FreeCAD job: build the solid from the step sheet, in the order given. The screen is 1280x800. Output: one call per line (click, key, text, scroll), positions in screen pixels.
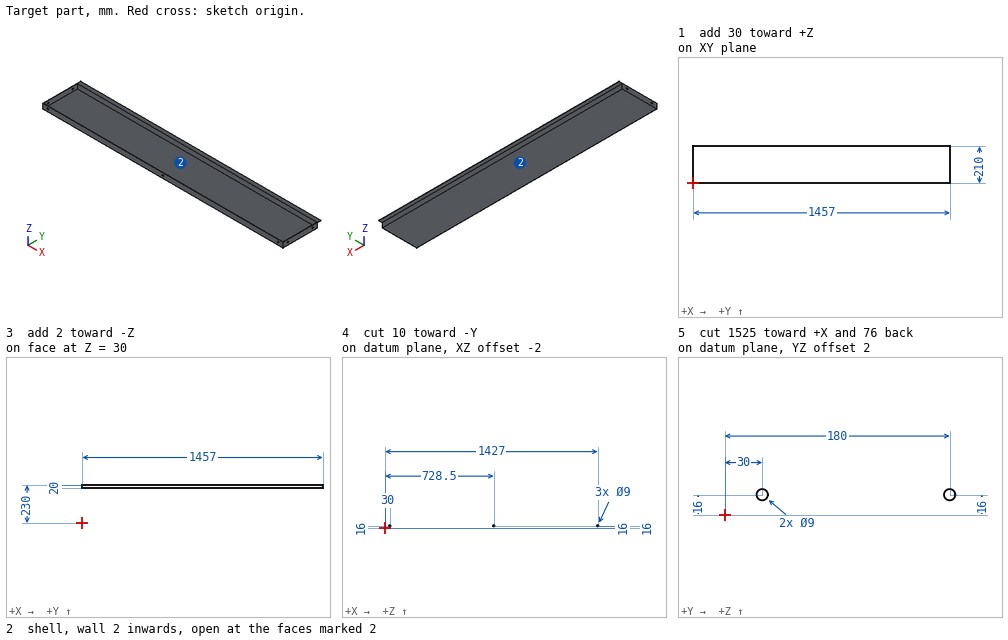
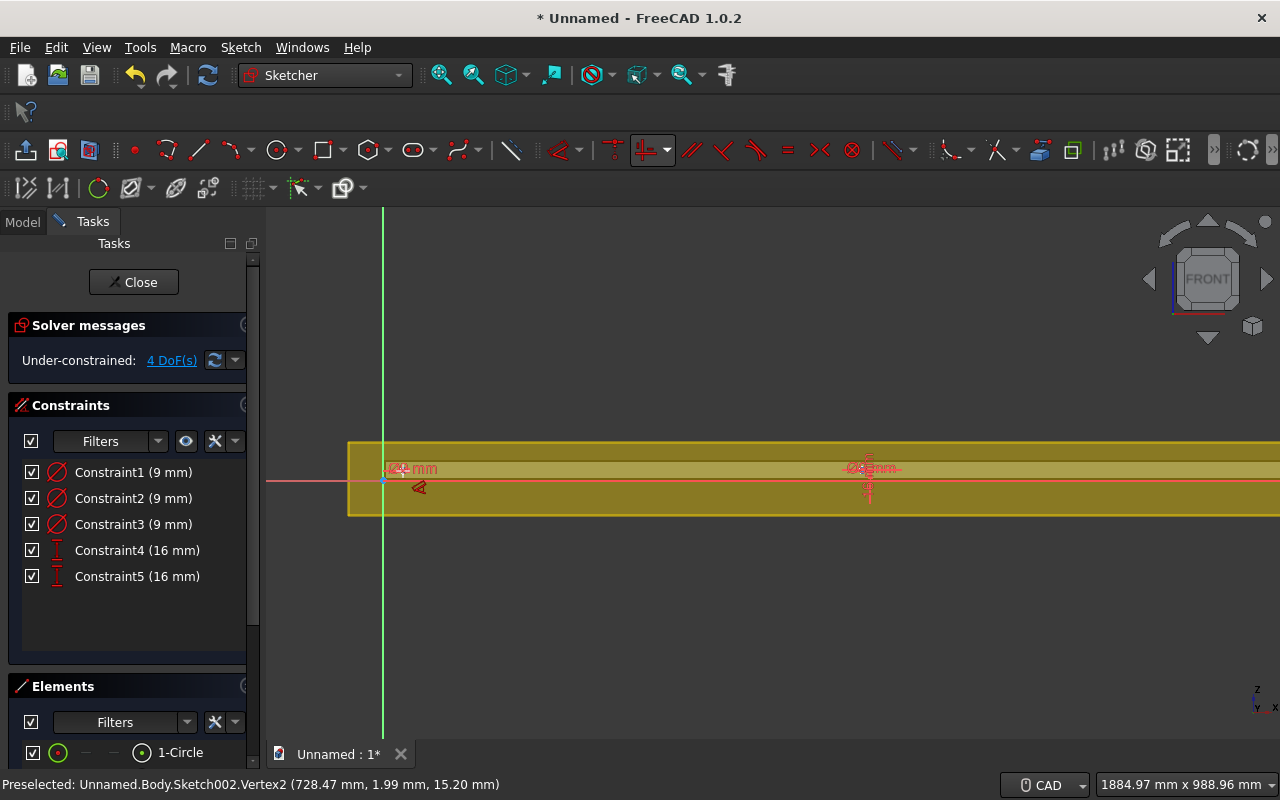
click(404, 470)
click(381, 526)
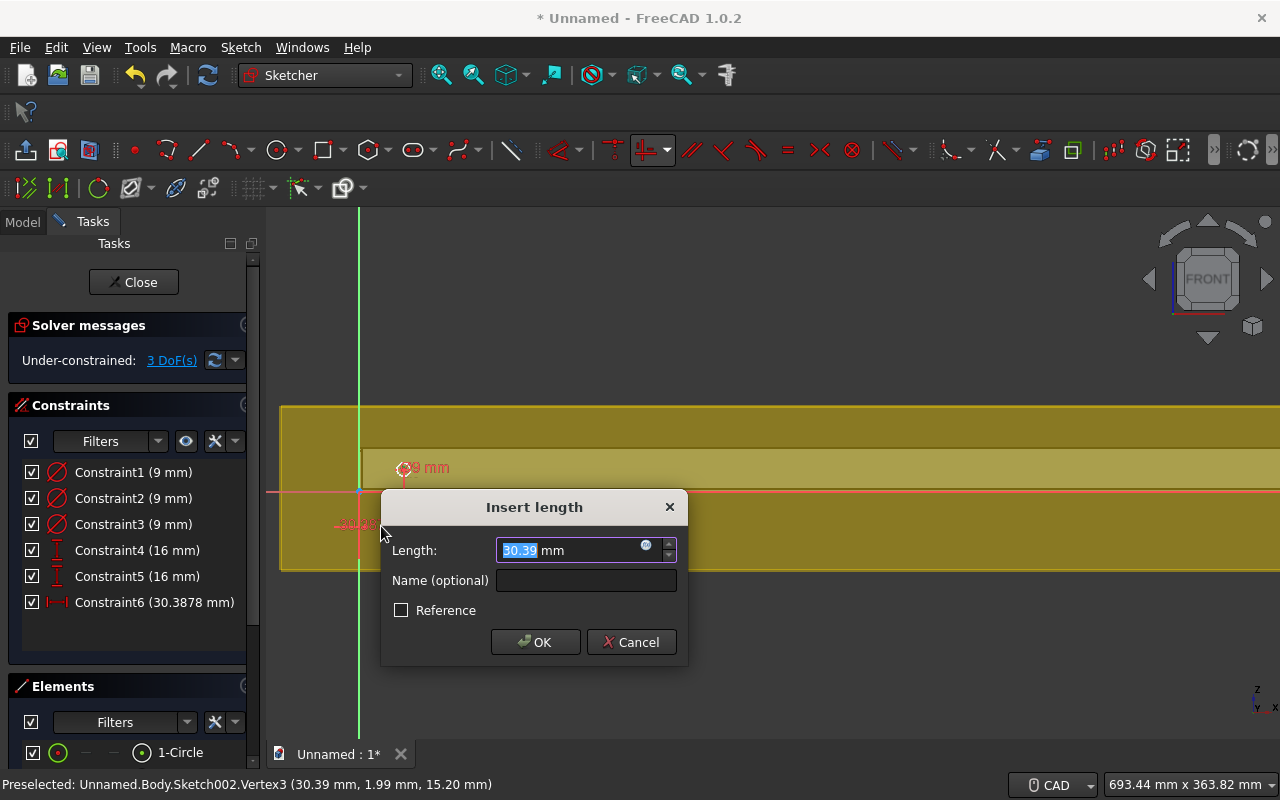
text(30)
key(Return)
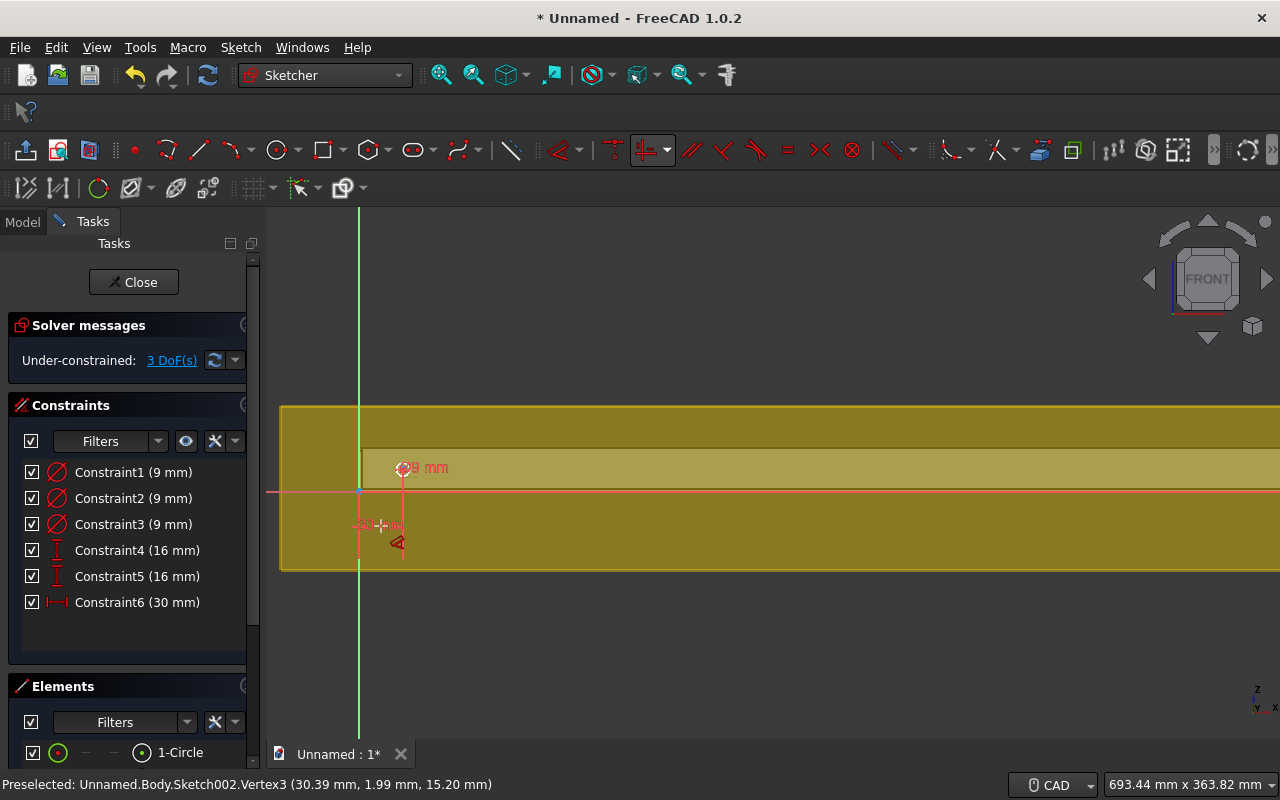
scroll(403, 470, up, 3)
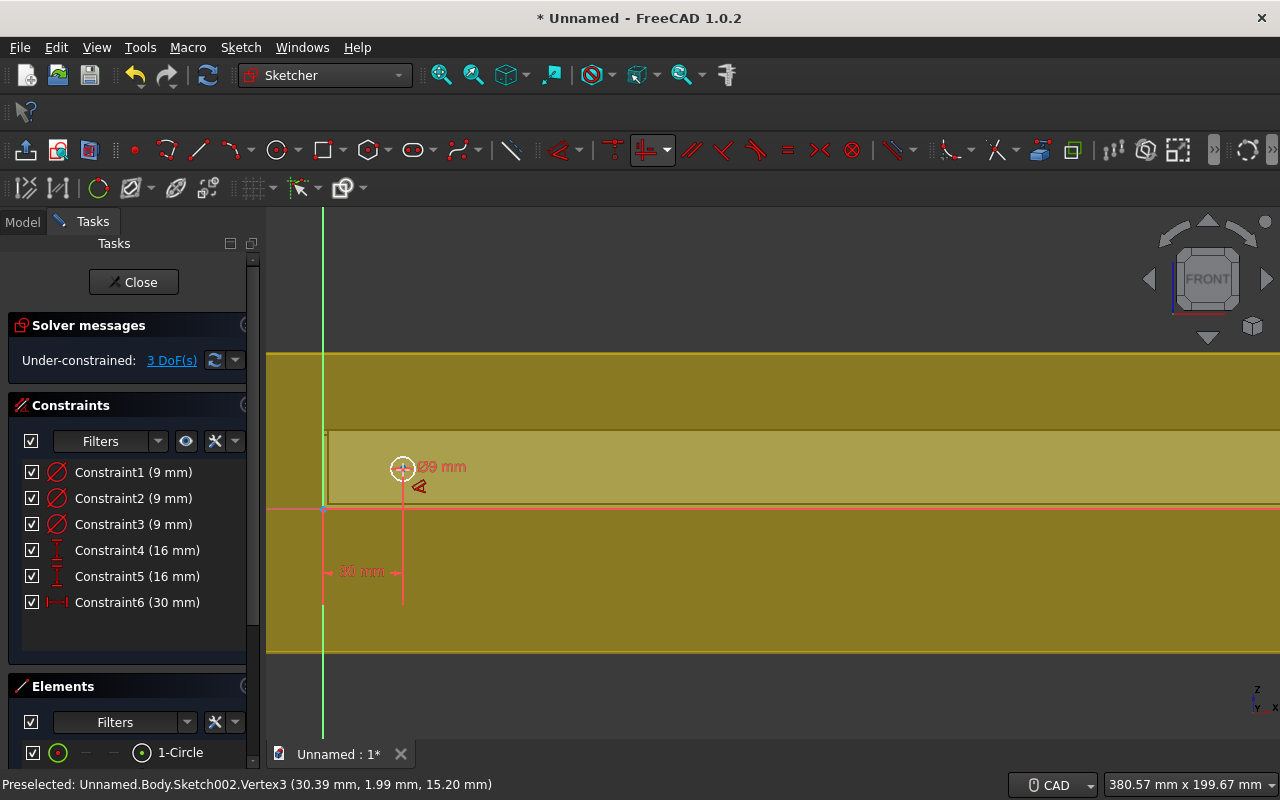
click(403, 469)
click(437, 489)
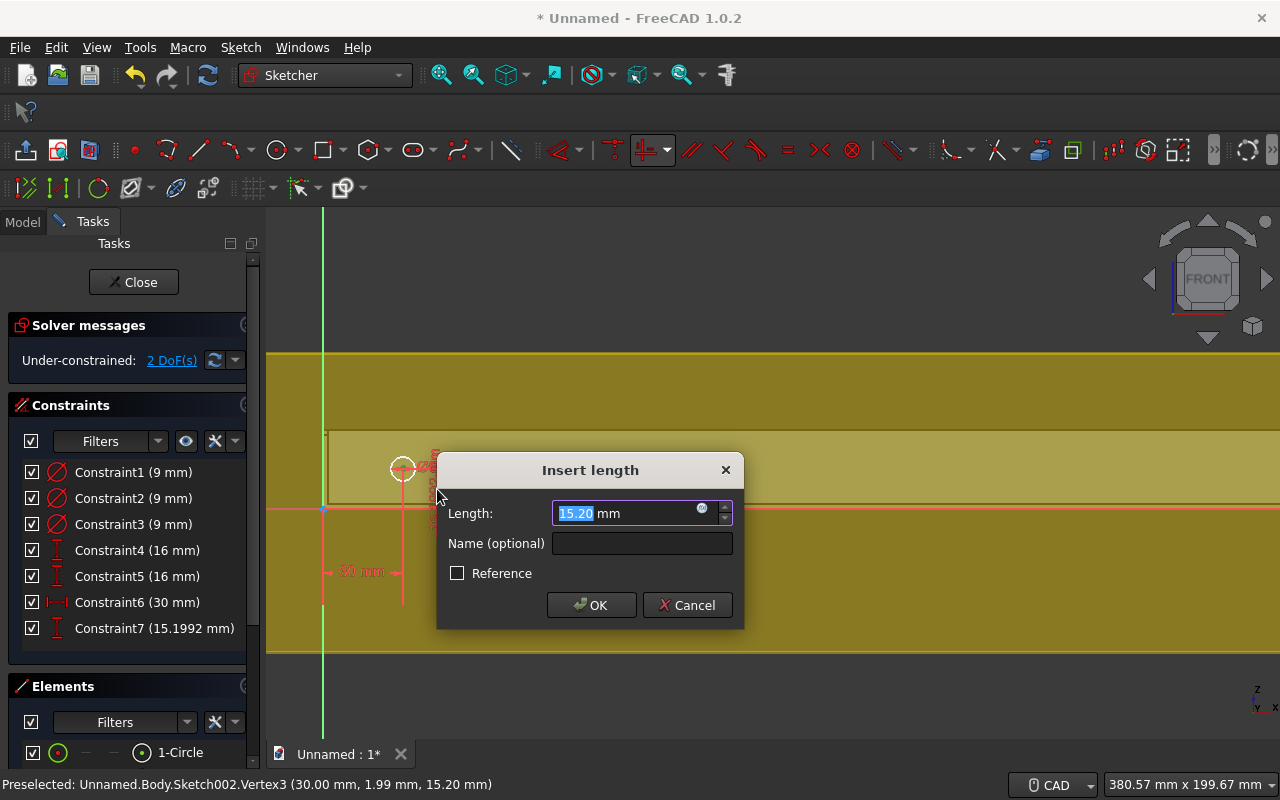
text(16)
key(Return)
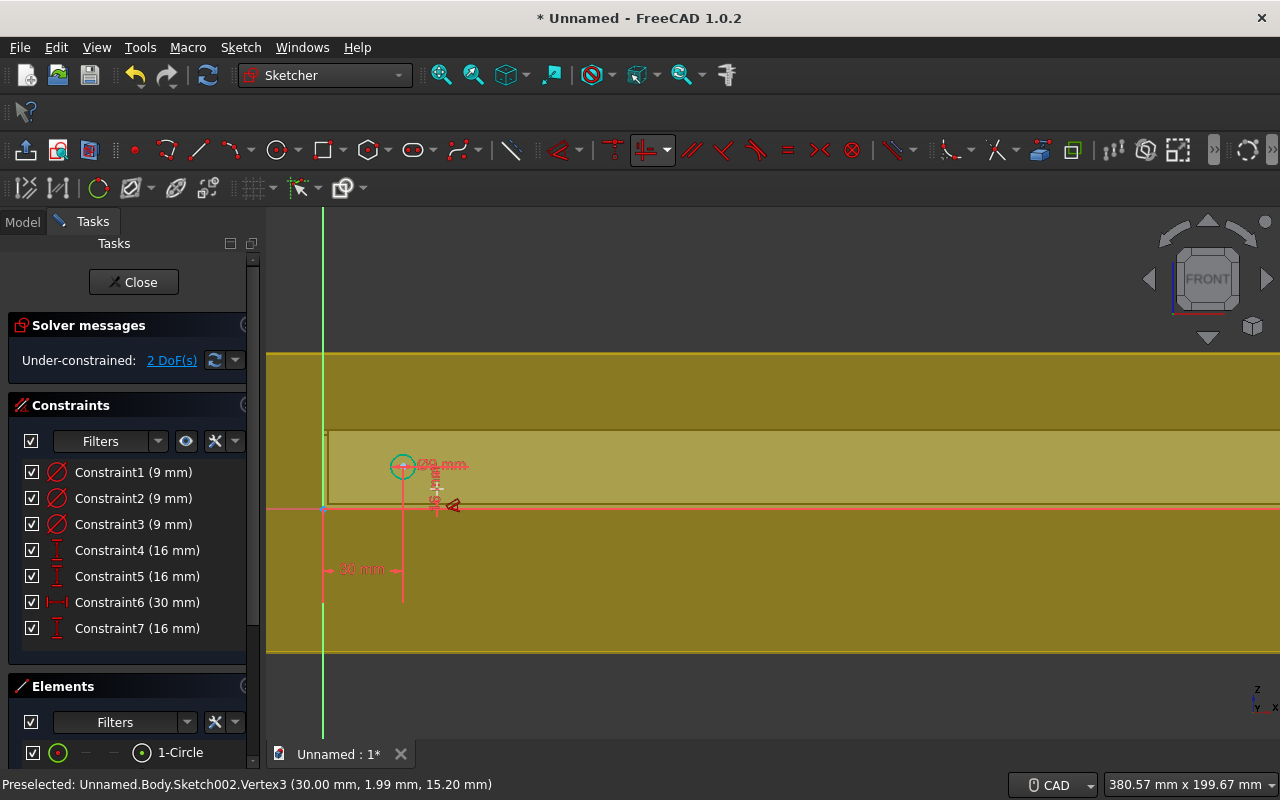
scroll(402, 471, down, 9)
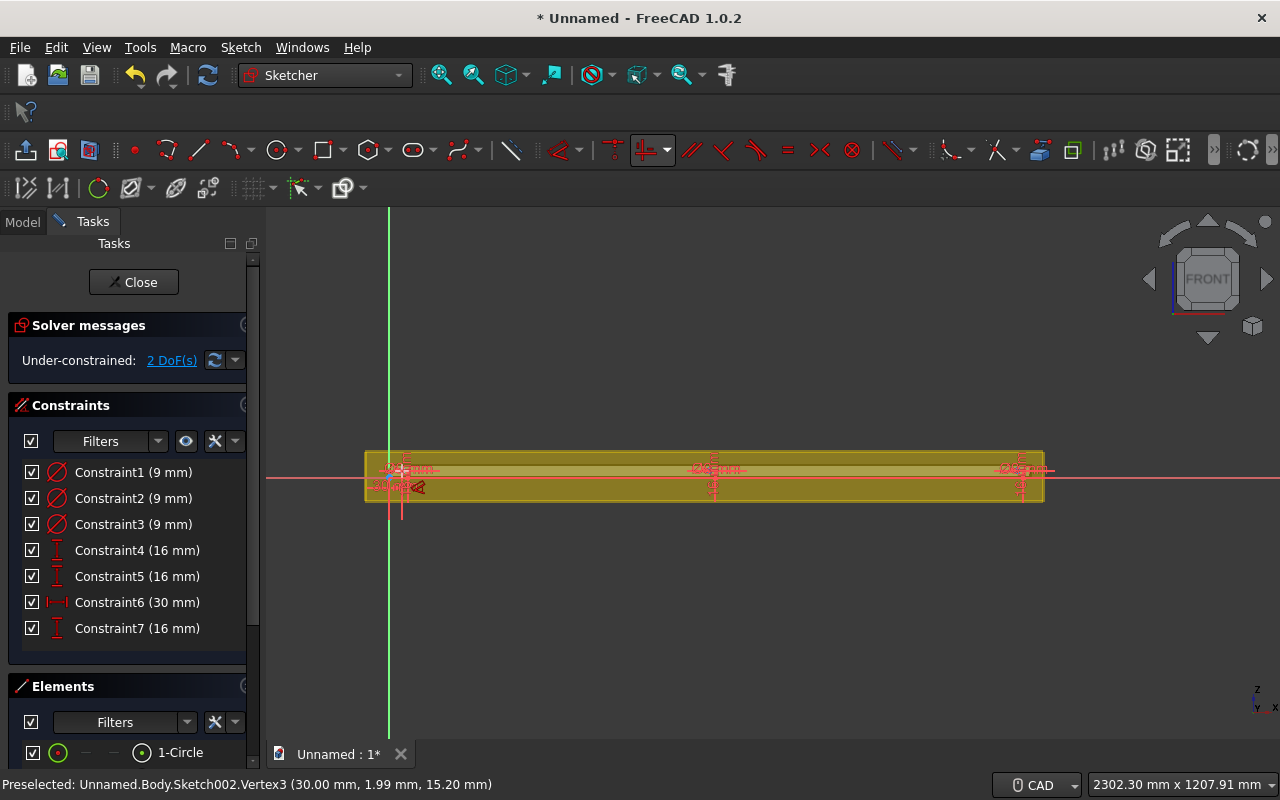
click(1017, 471)
click(703, 512)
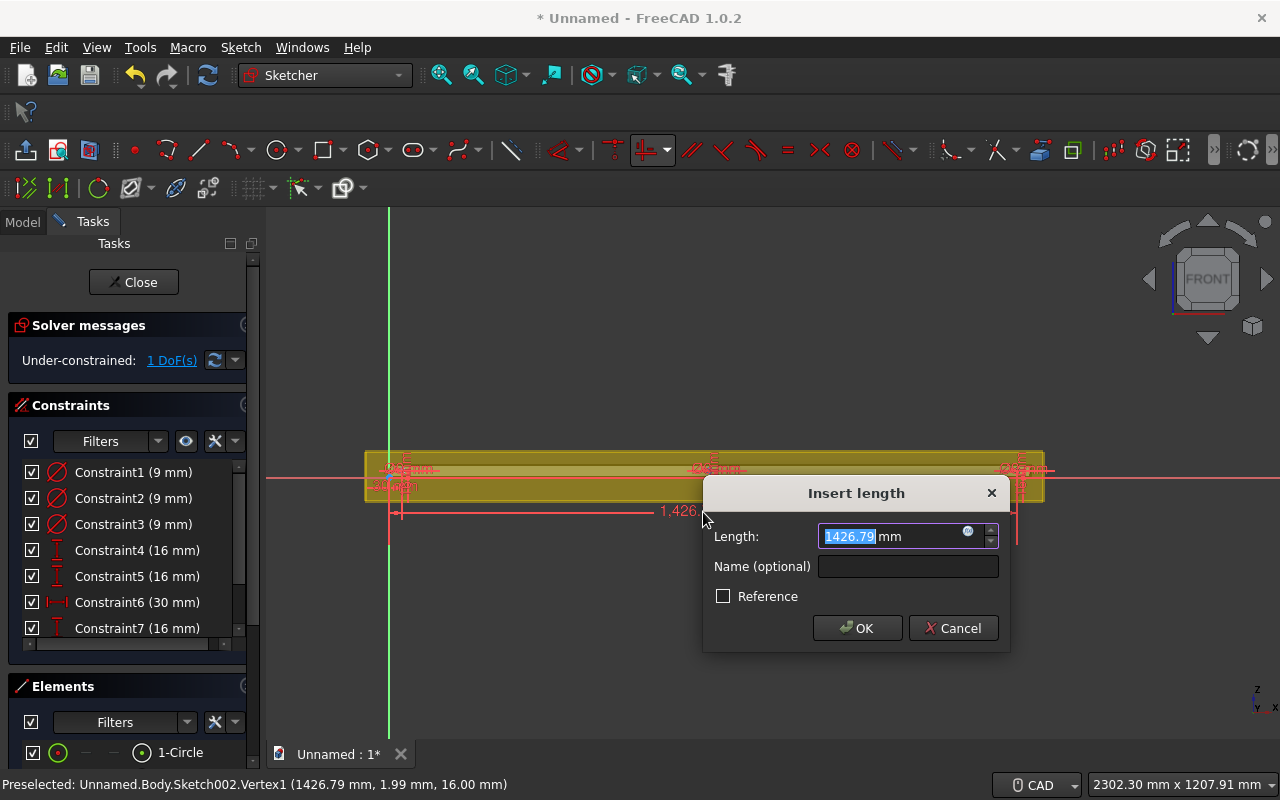
text(1427)
key(Return)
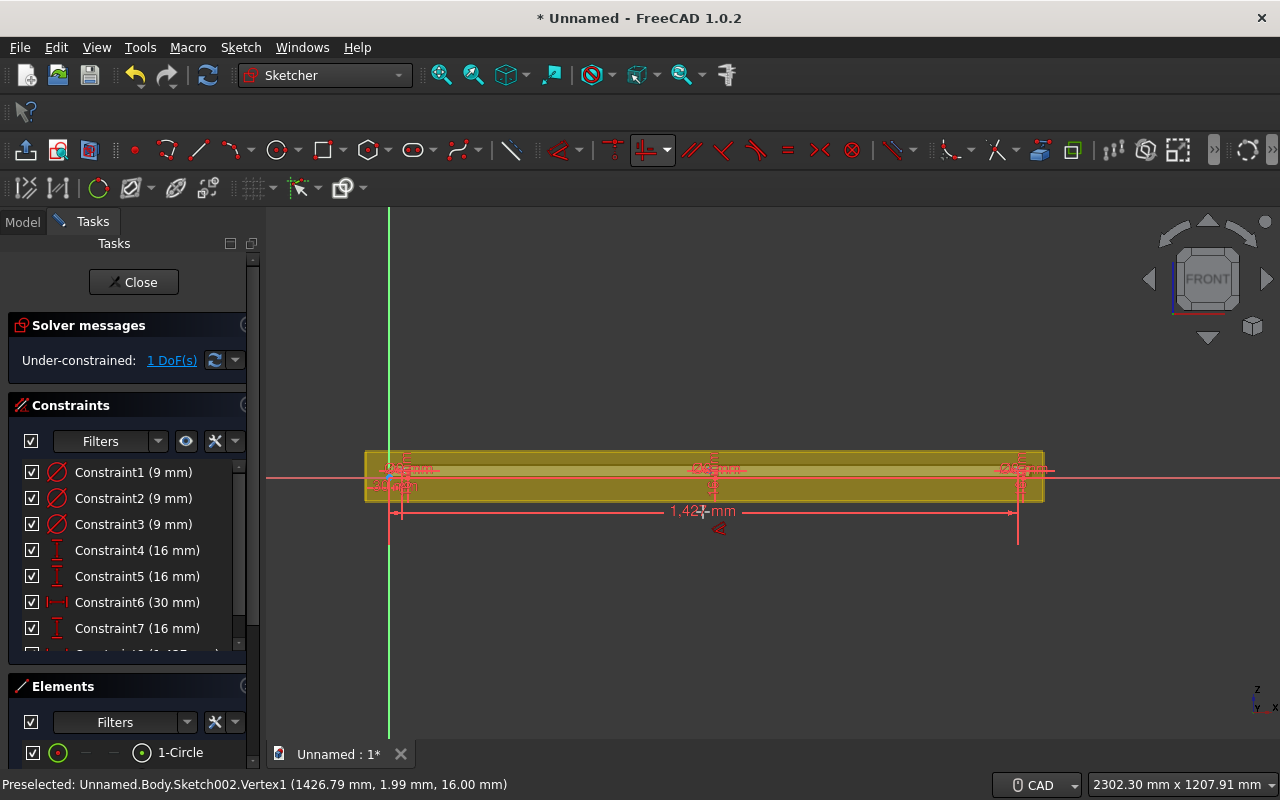
click(710, 471)
click(549, 512)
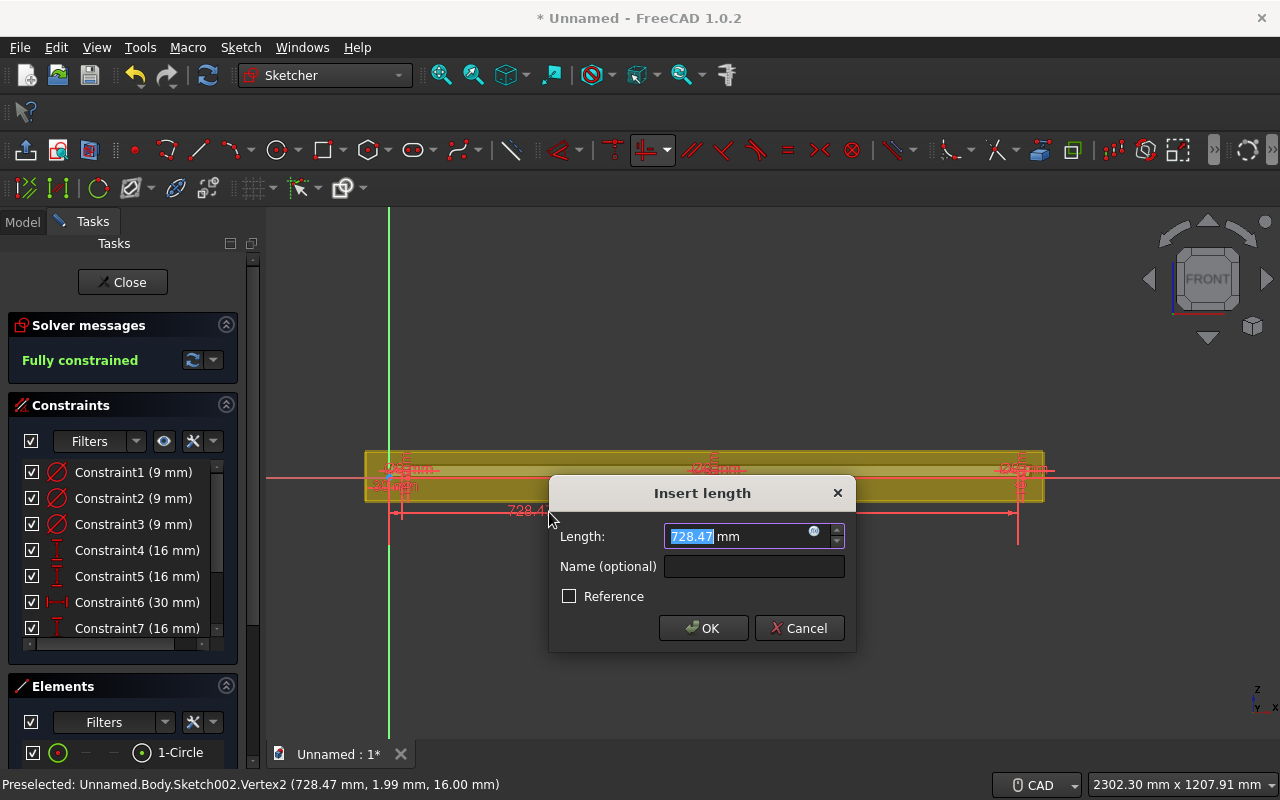
text(728.5)
key(Return)
key(Escape)